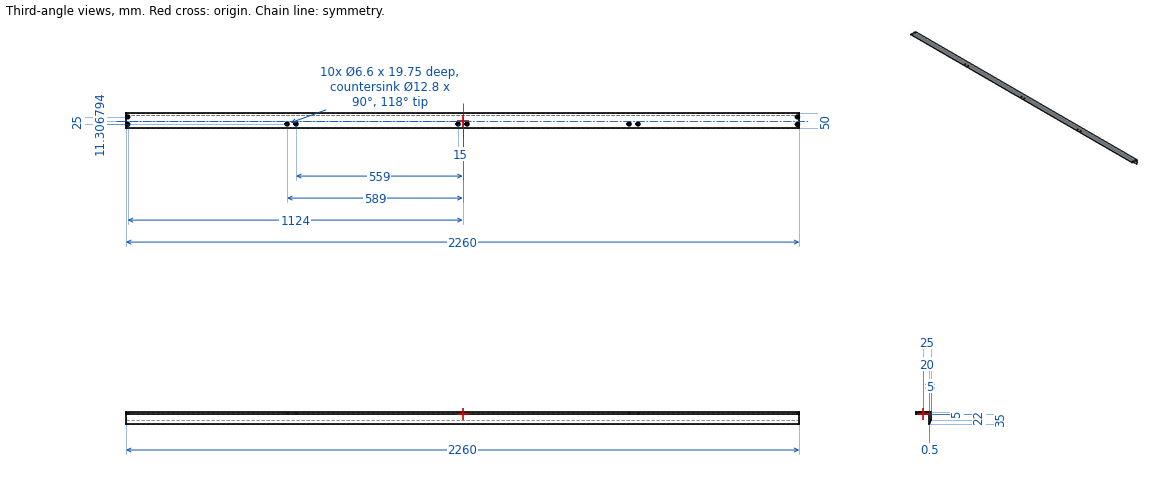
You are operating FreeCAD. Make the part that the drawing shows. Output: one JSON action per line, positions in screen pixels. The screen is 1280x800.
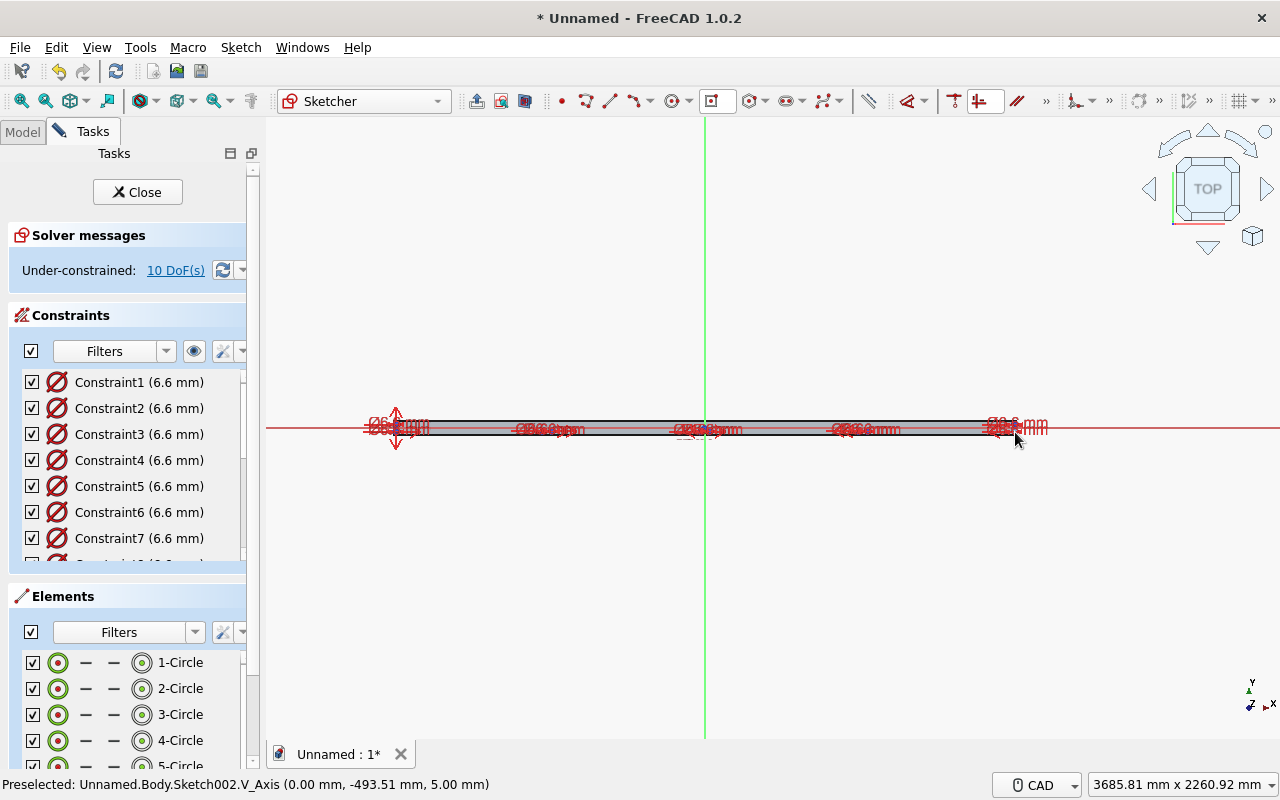
{"action": "scroll", "coordinate": [396, 425], "scroll_direction": "up", "scroll_amount": 3}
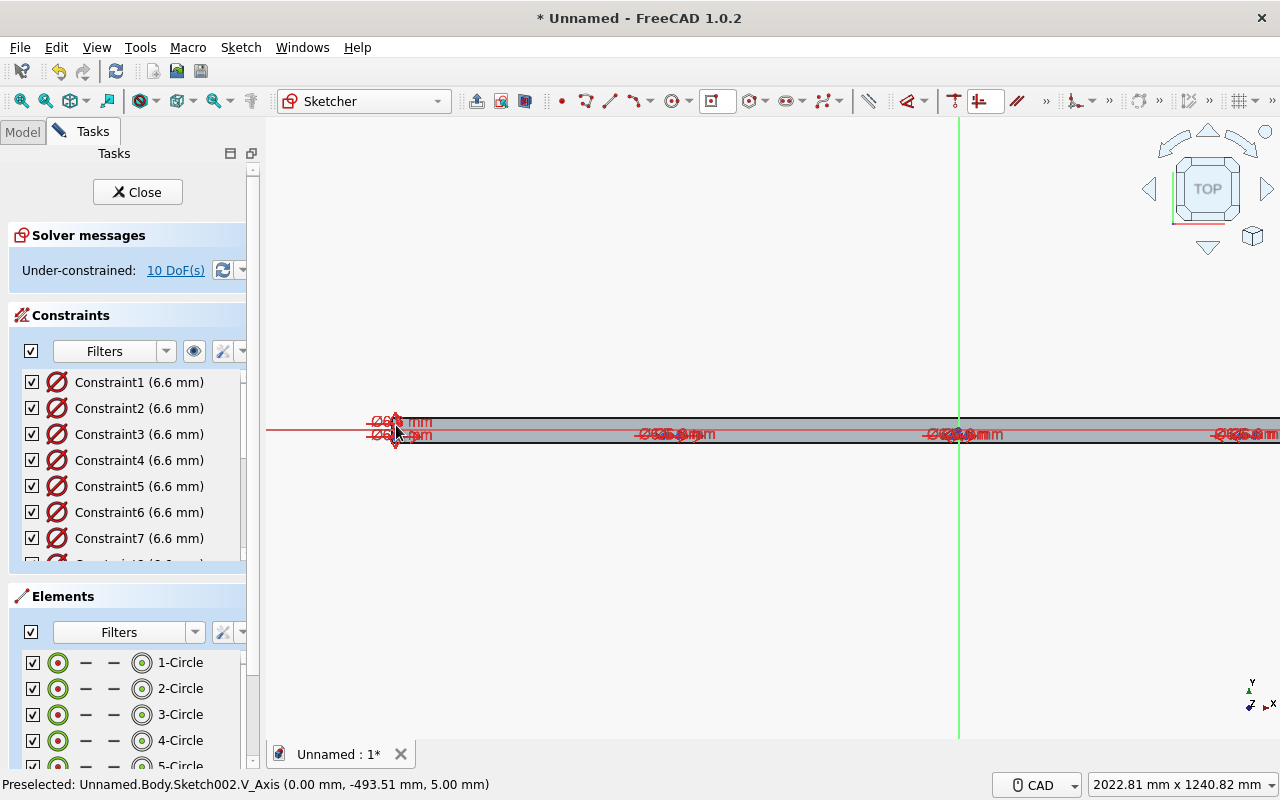
{"action": "left_click", "coordinate": [396, 424]}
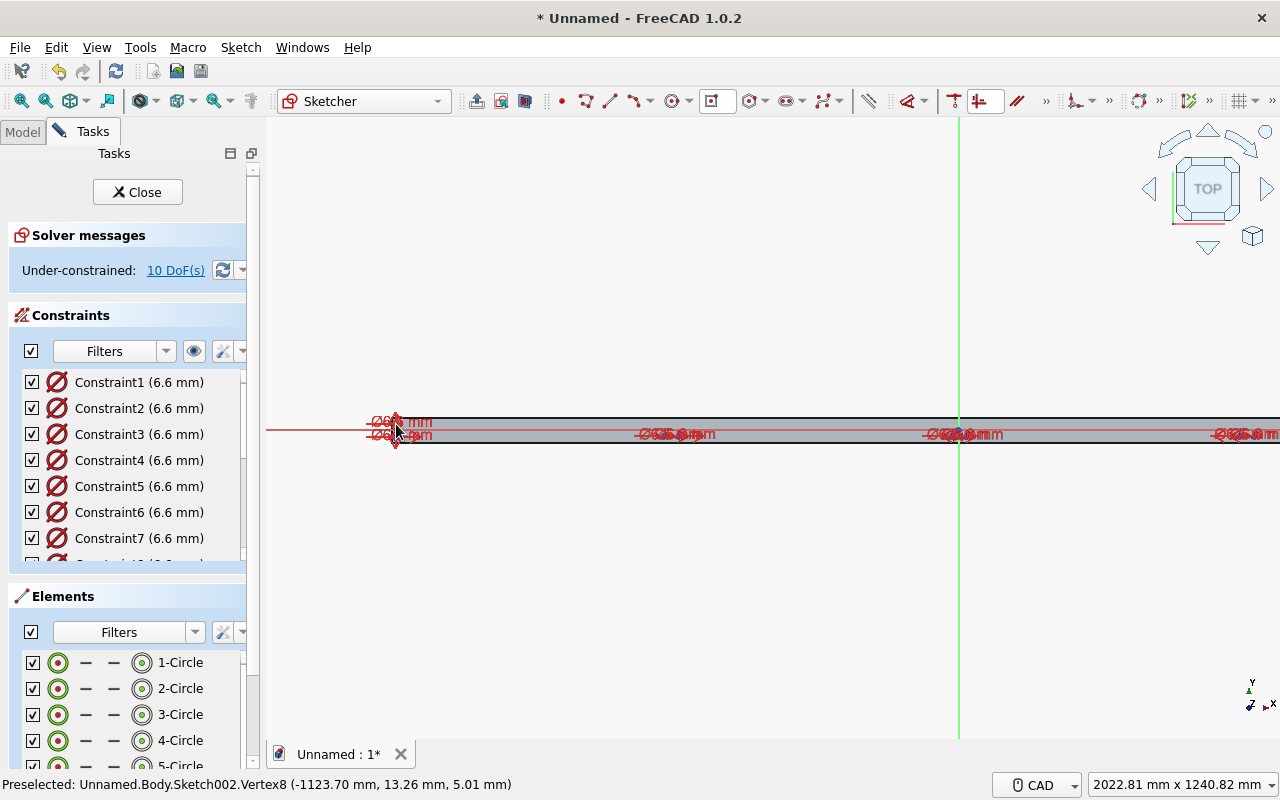
{"action": "scroll", "coordinate": [395, 425], "scroll_direction": "down", "scroll_amount": 3}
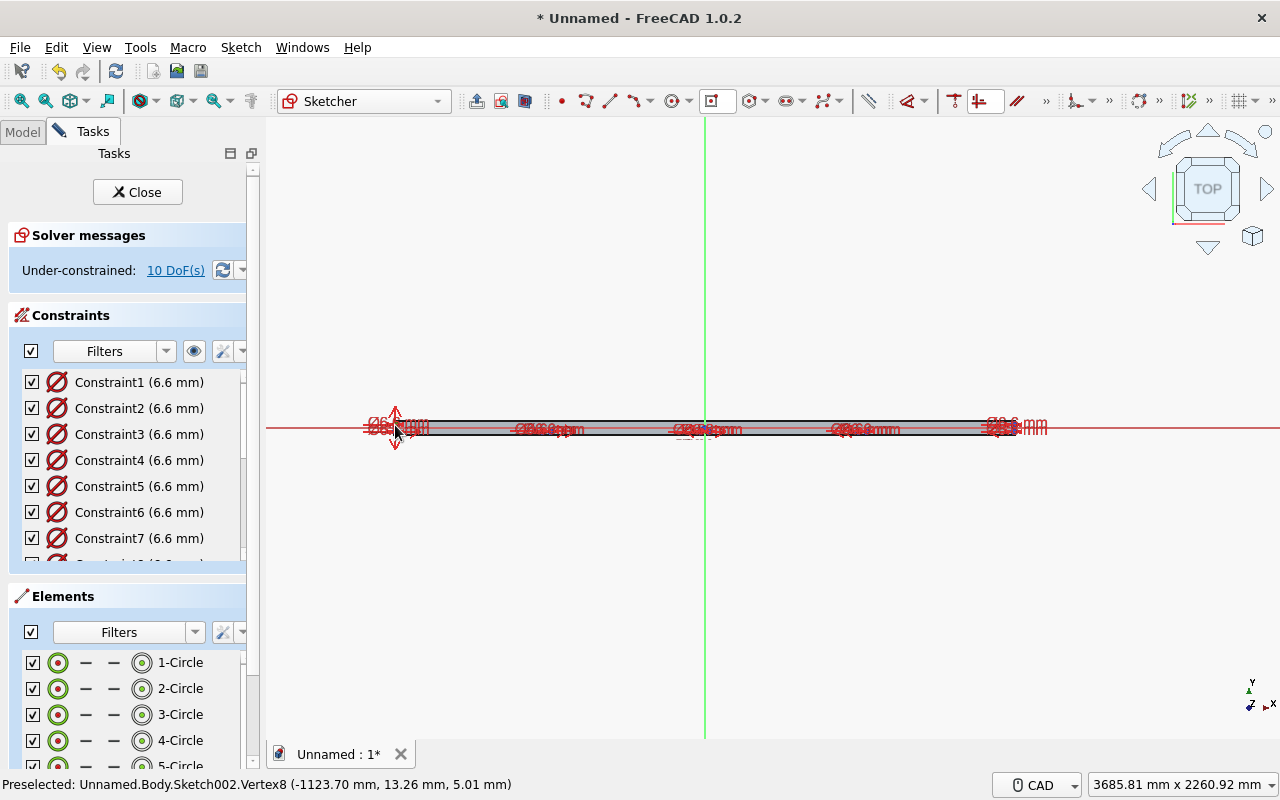
{"action": "scroll", "coordinate": [1014, 425], "scroll_direction": "up", "scroll_amount": 3}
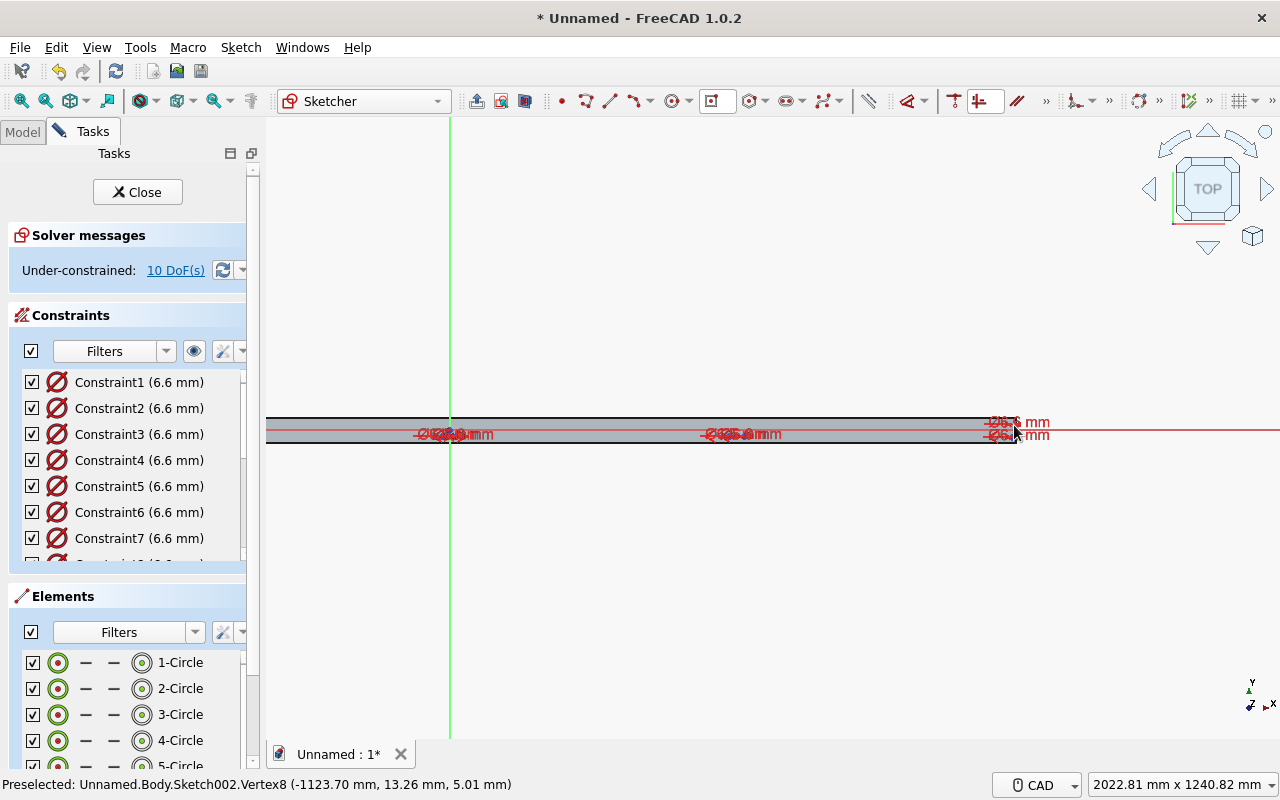
{"action": "left_click", "coordinate": [1013, 424]}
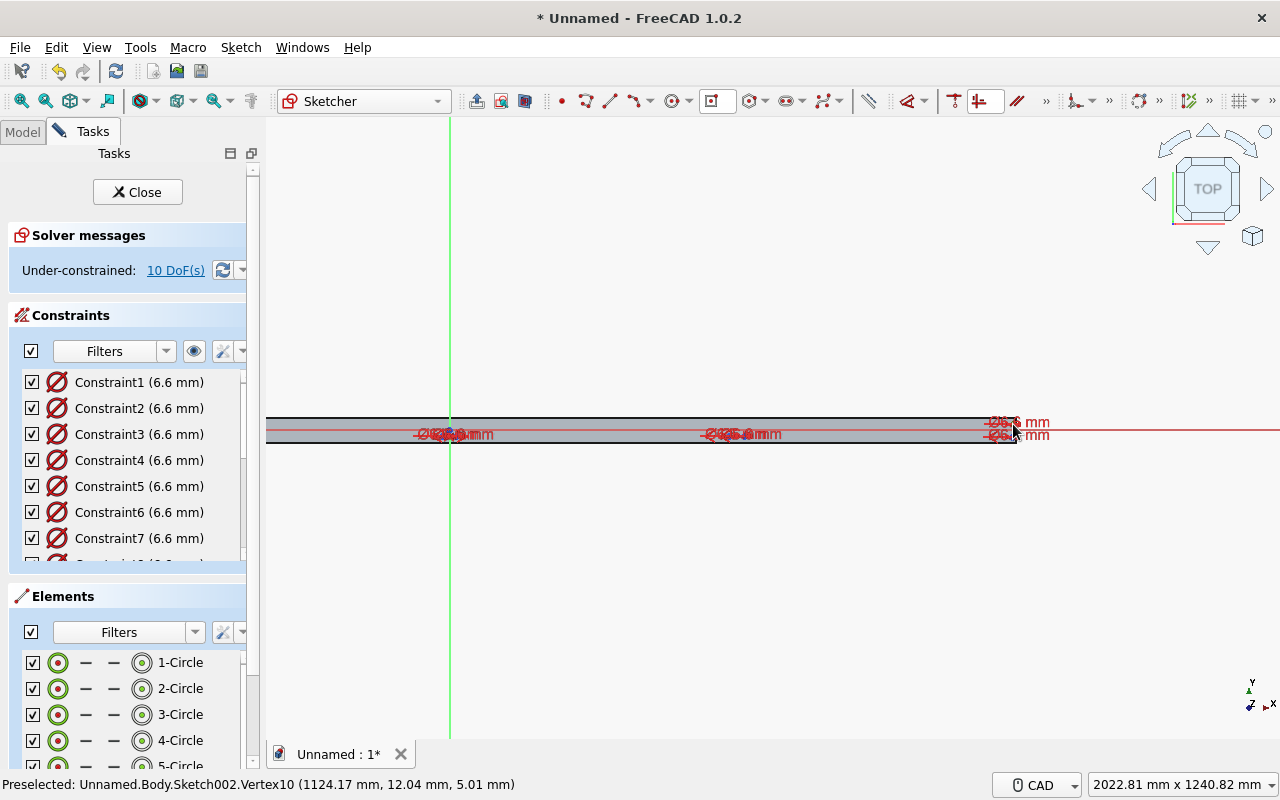
{"action": "left_click", "coordinate": [450, 671]}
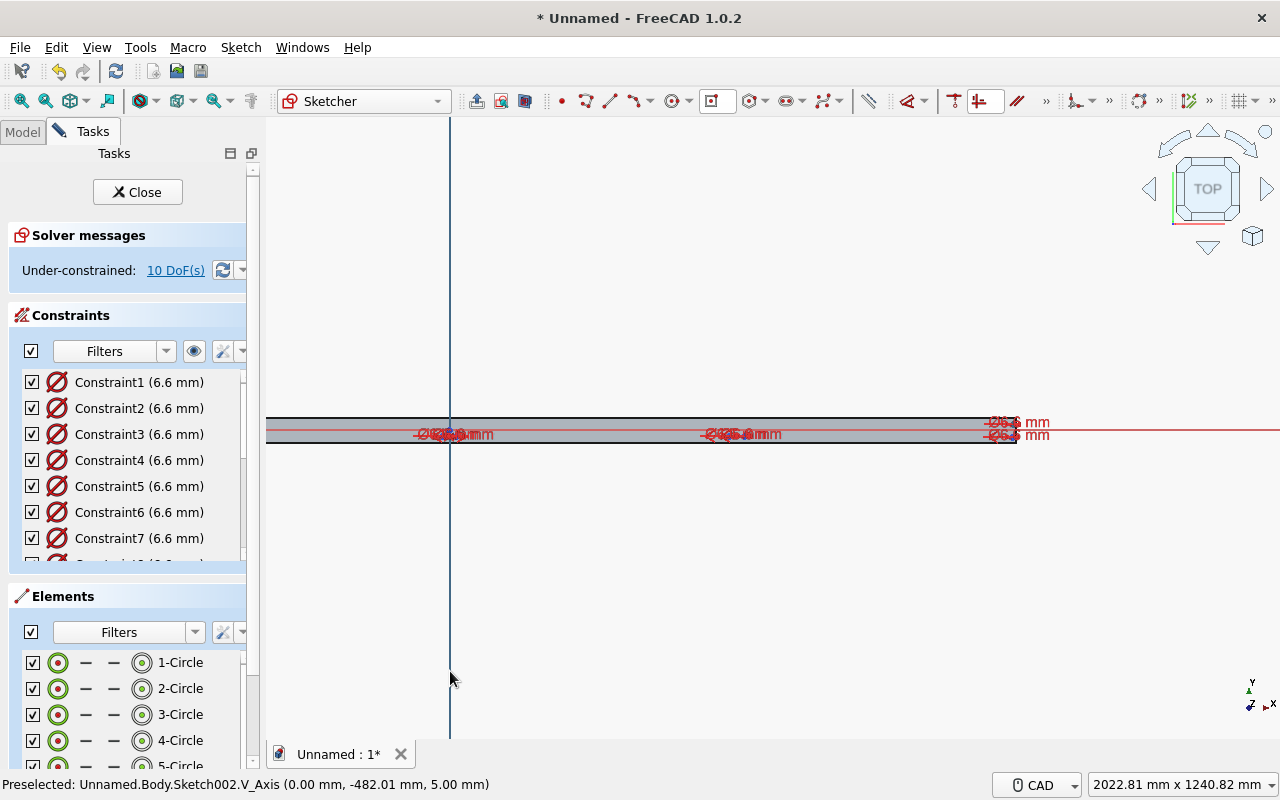
{"action": "key", "text": "s"}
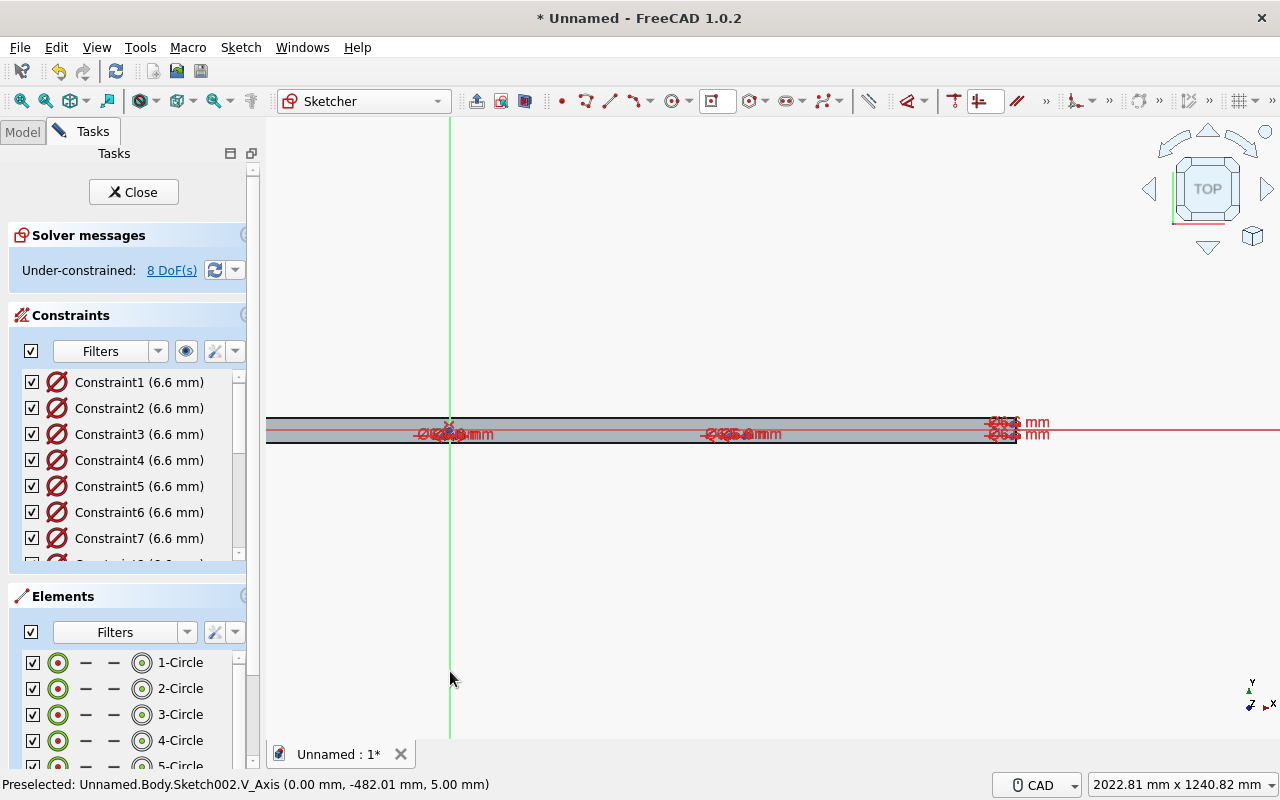
{"action": "left_click", "coordinate": [908, 102]}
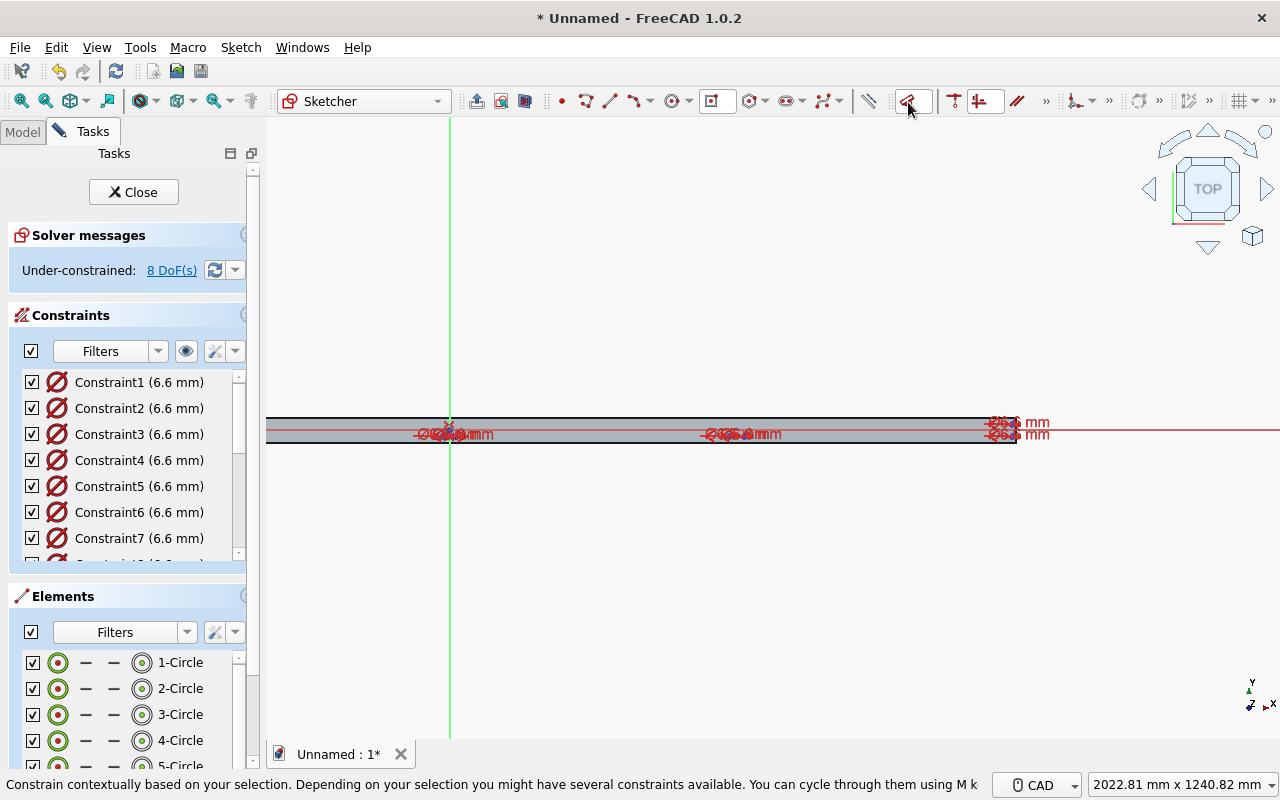
{"action": "scroll", "coordinate": [442, 436], "scroll_direction": "up", "scroll_amount": 9}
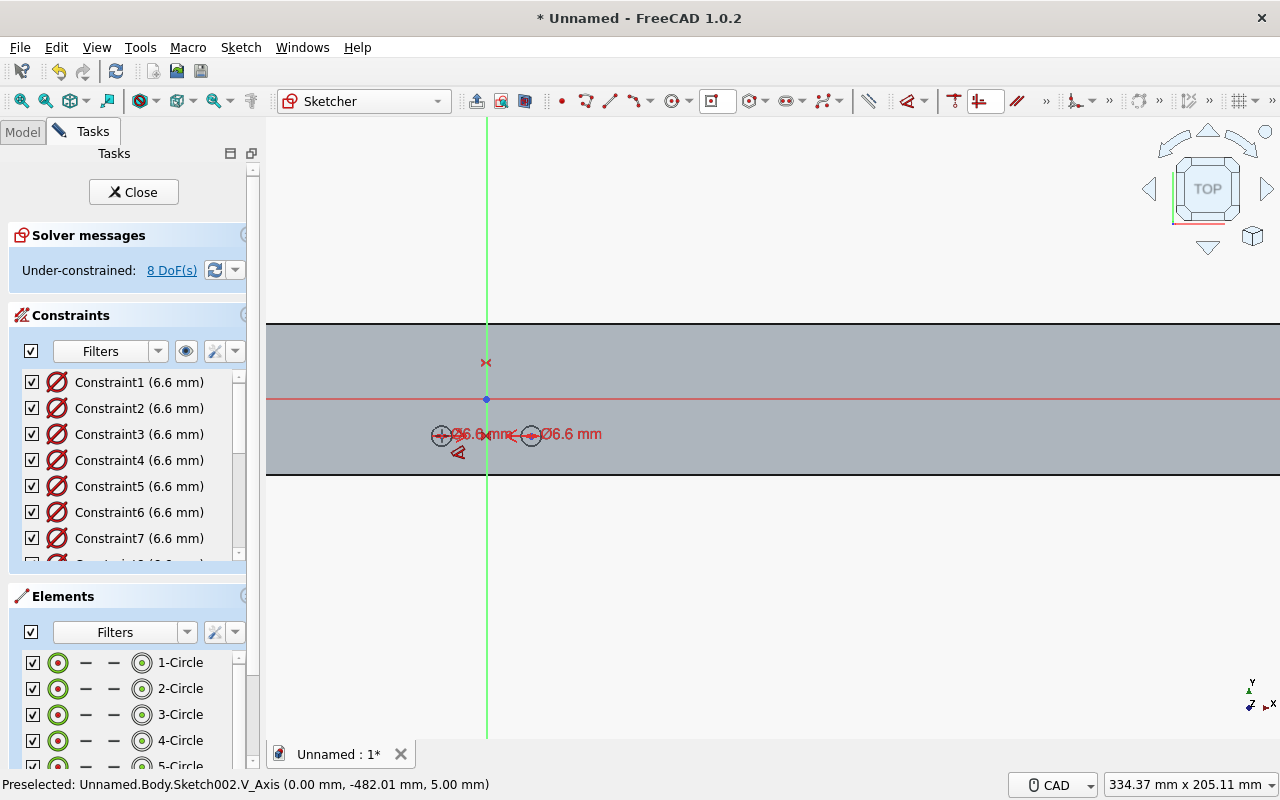
{"action": "left_click", "coordinate": [442, 436]}
{"action": "left_click", "coordinate": [464, 470]}